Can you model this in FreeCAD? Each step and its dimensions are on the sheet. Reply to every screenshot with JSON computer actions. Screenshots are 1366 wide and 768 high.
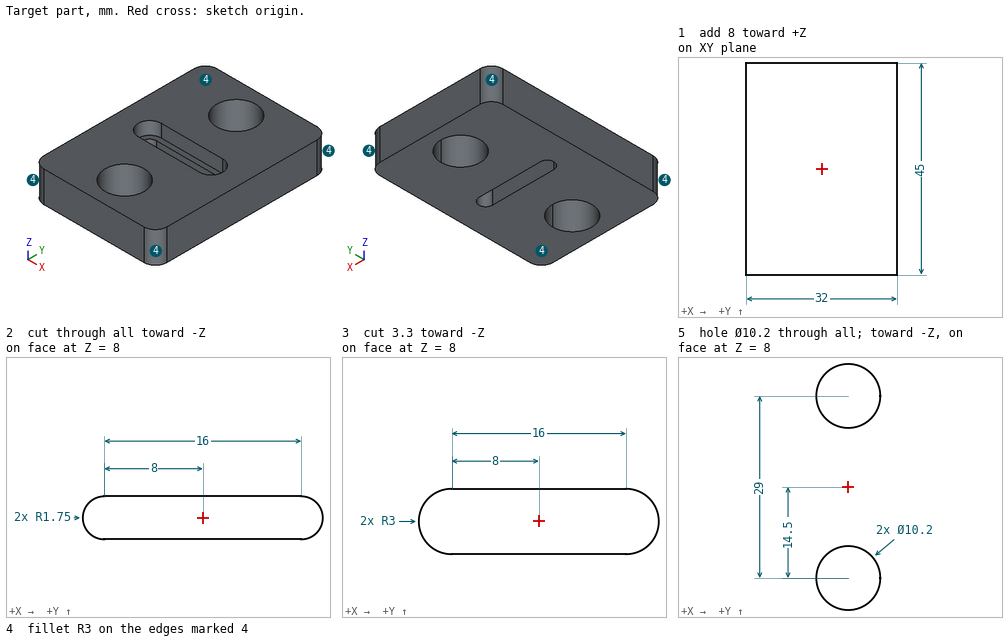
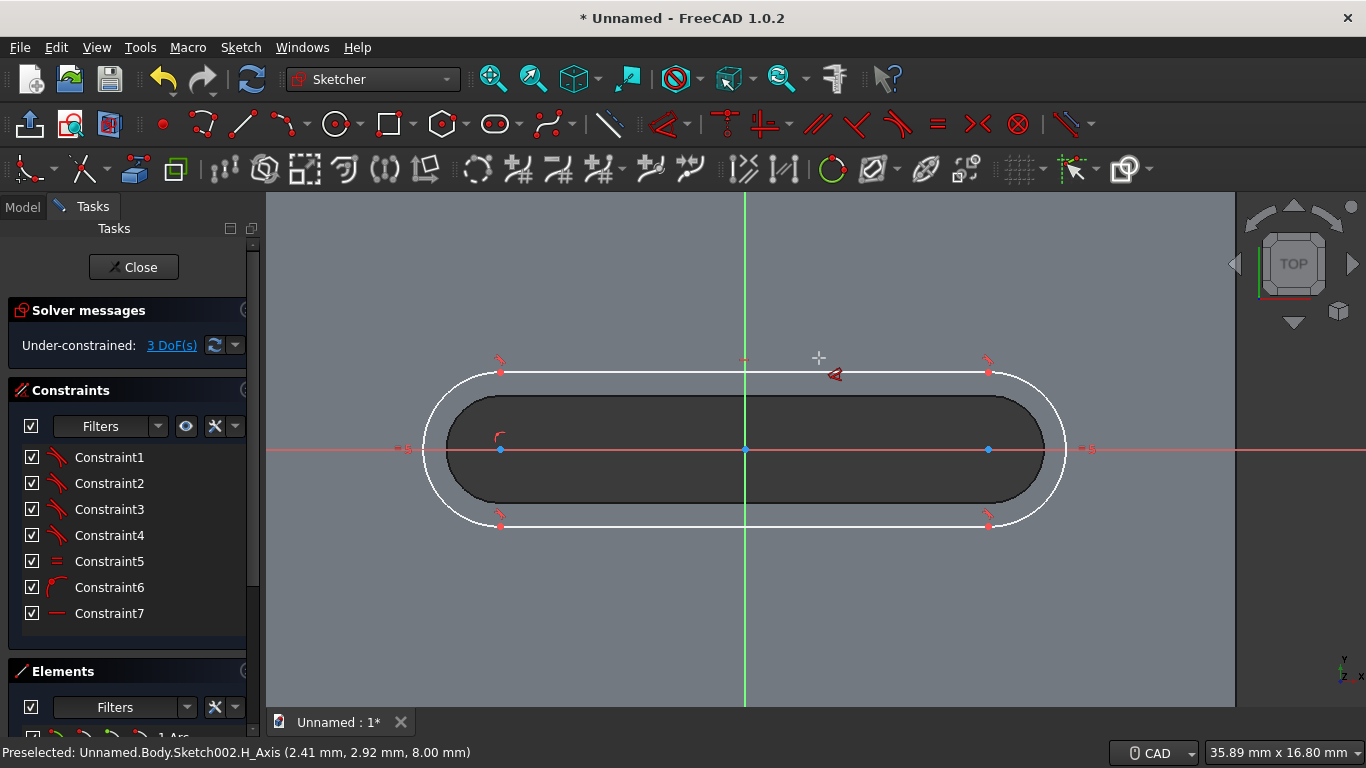
{"action": "left_click", "coordinate": [438, 404]}
{"action": "left_click", "coordinate": [412, 385]}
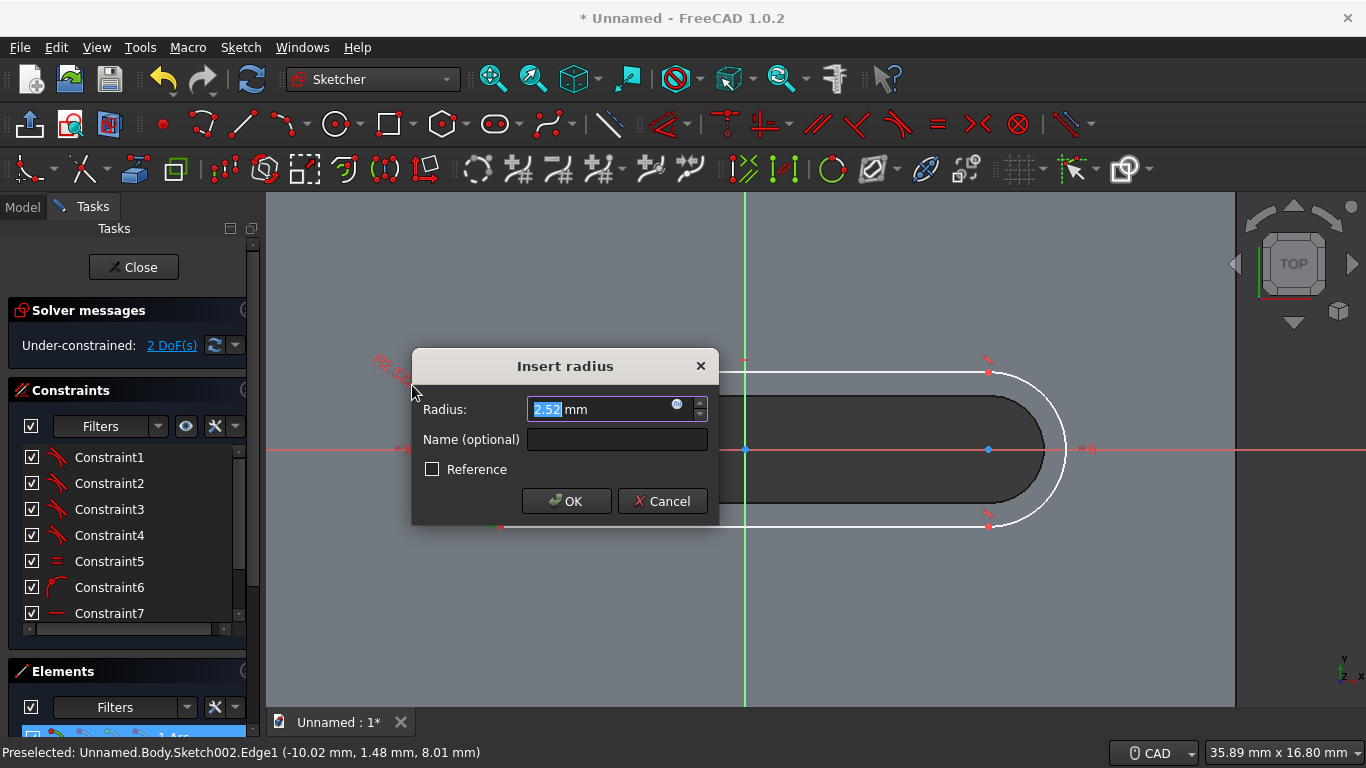
{"action": "type", "text": "3"}
{"action": "key", "text": "Return"}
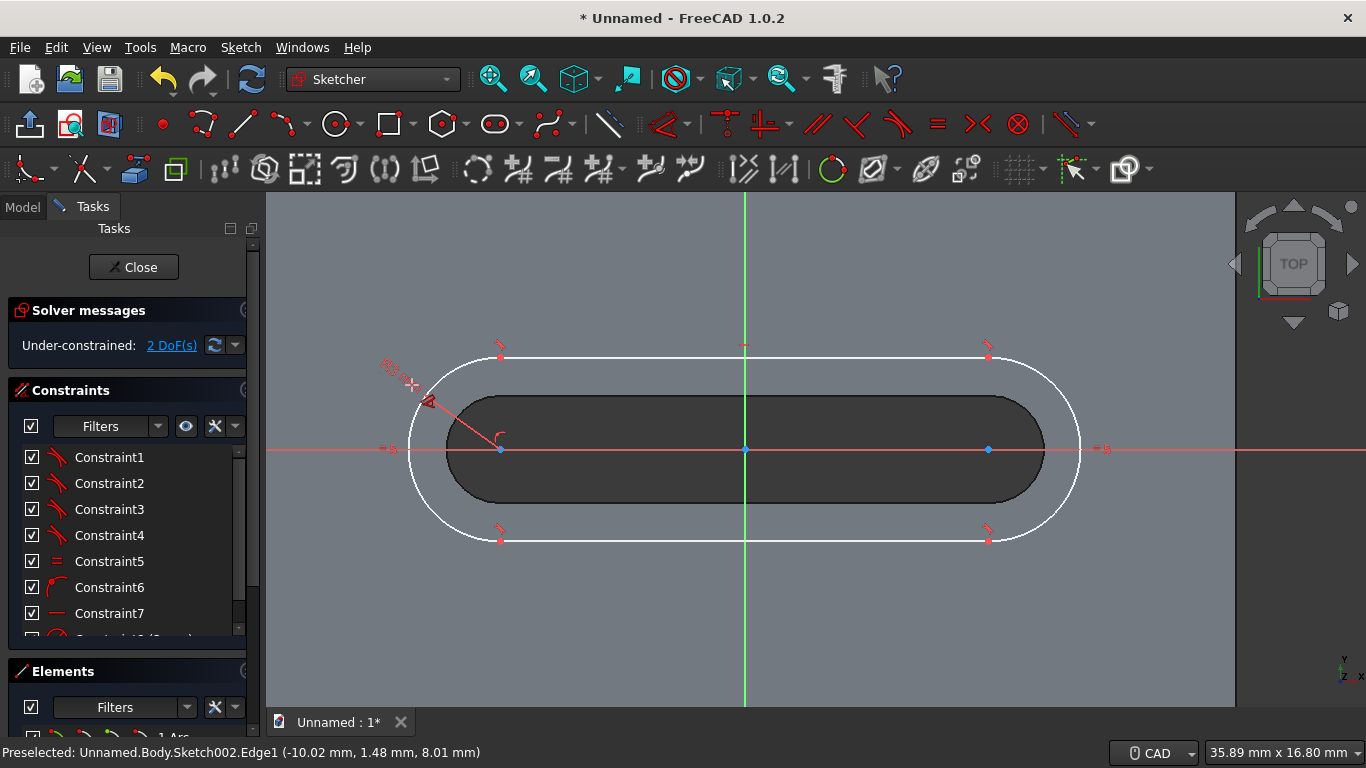
{"action": "left_click", "coordinate": [647, 358]}
{"action": "left_click", "coordinate": [632, 324]}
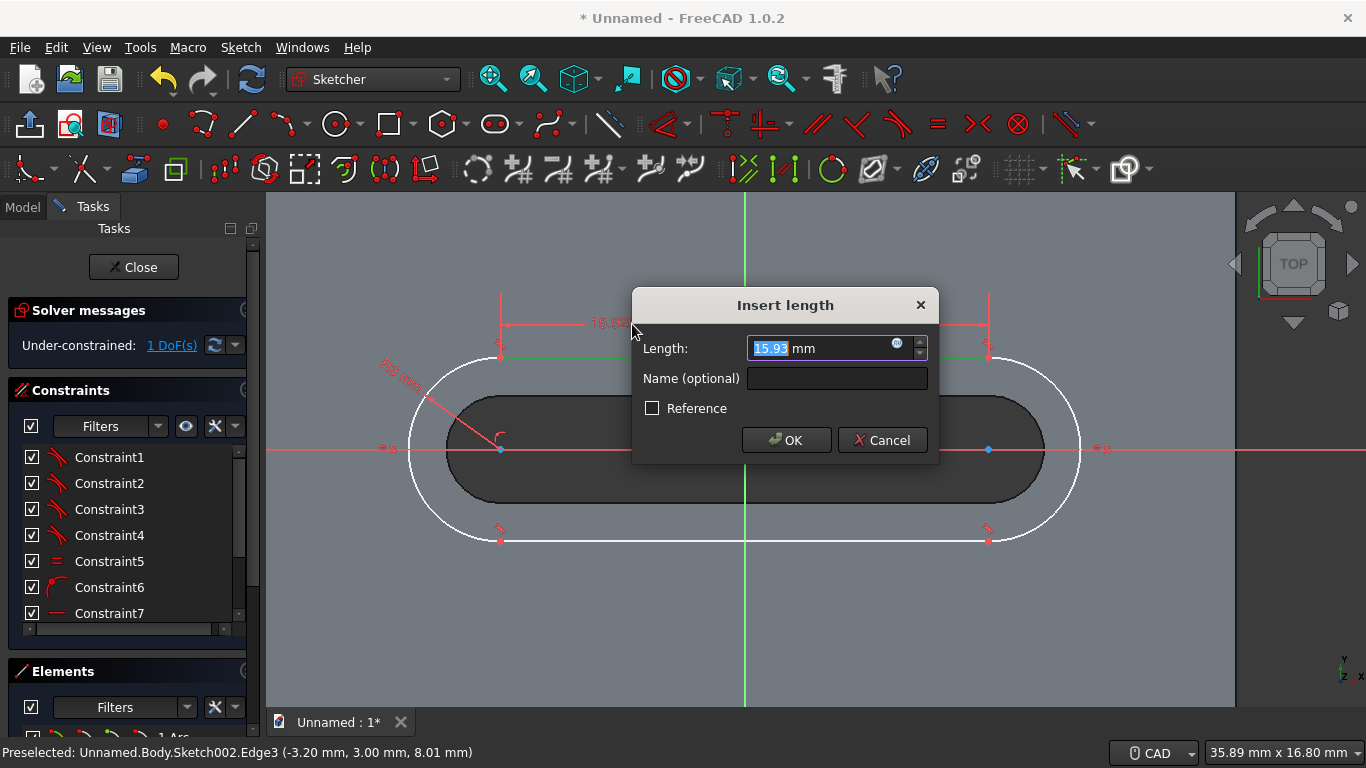
{"action": "type", "text": "16"}
{"action": "key", "text": "Return"}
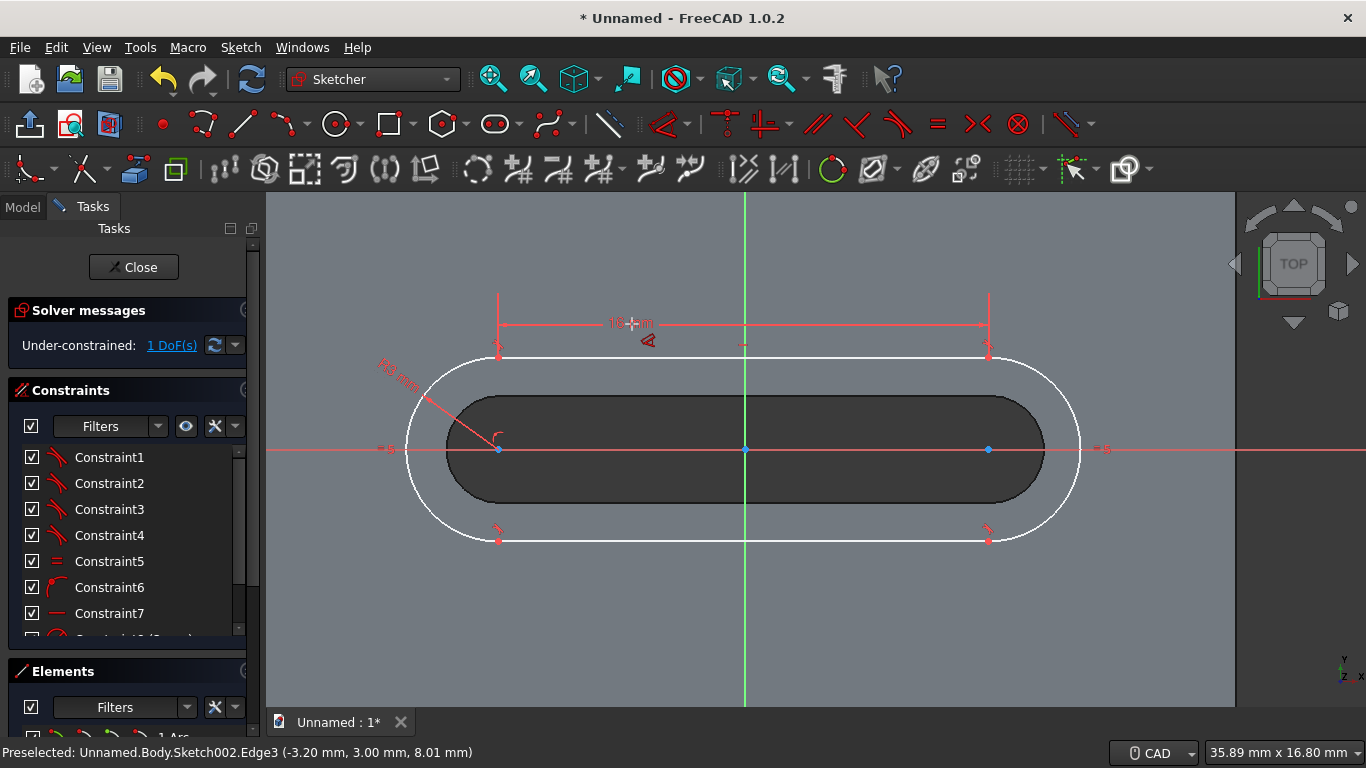
{"action": "left_click", "coordinate": [498, 358]}
{"action": "left_click", "coordinate": [535, 324]}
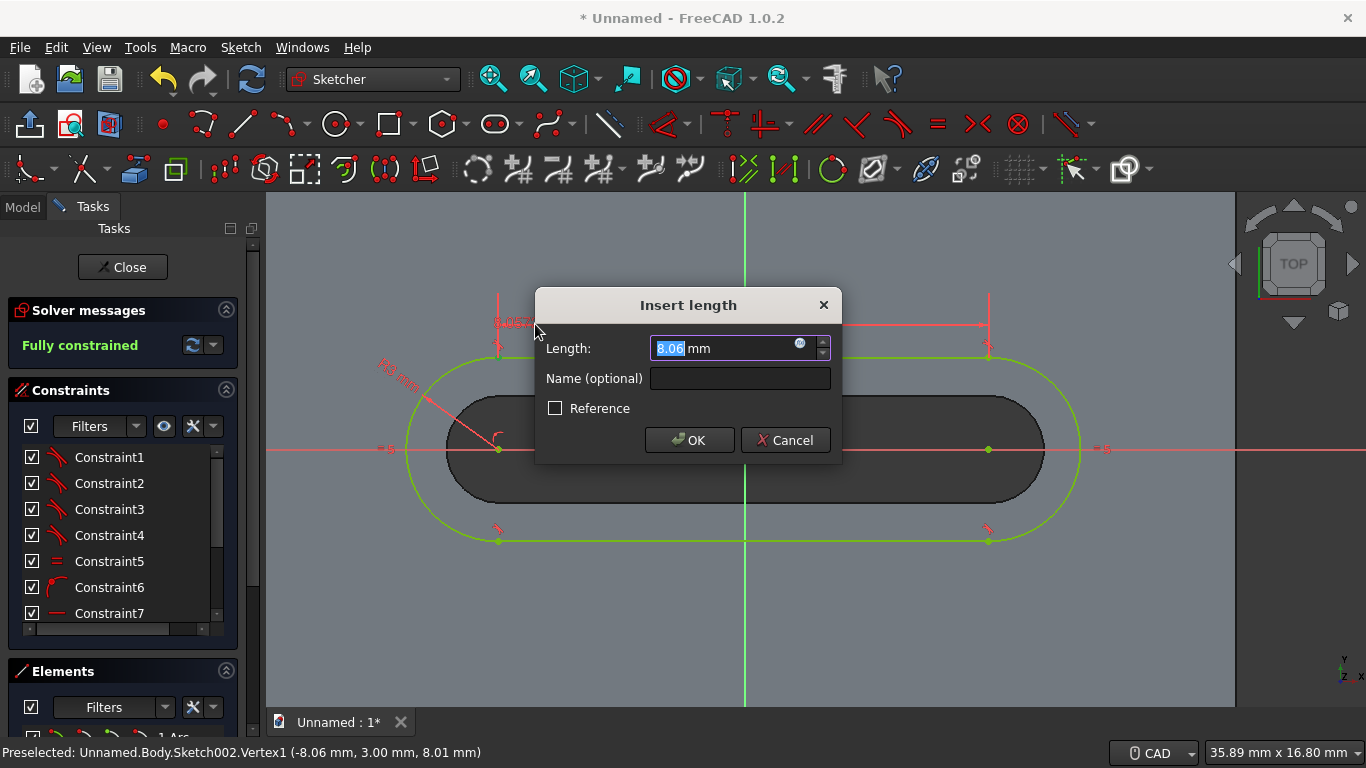
{"action": "type", "text": "8"}
{"action": "key", "text": "Return"}
{"action": "key", "text": "Escape"}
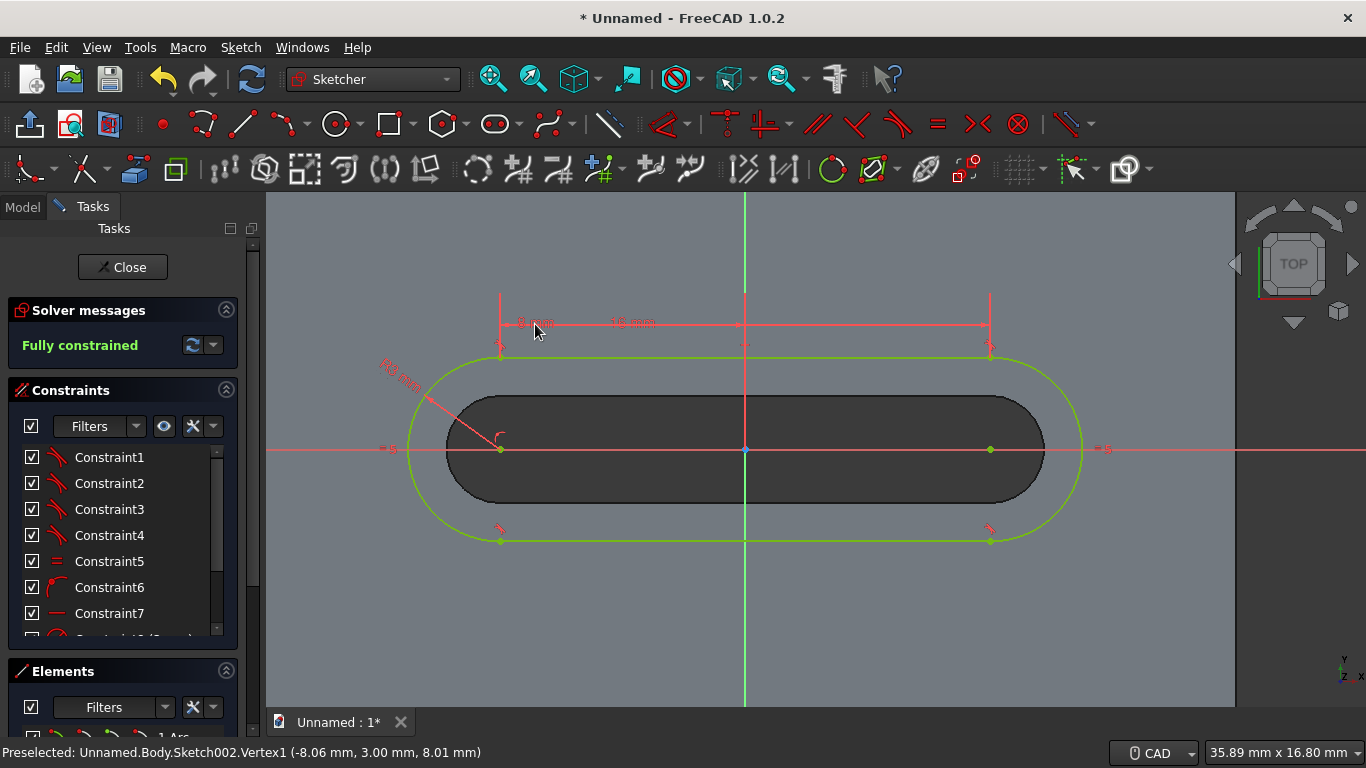
{"action": "left_click", "coordinate": [123, 267]}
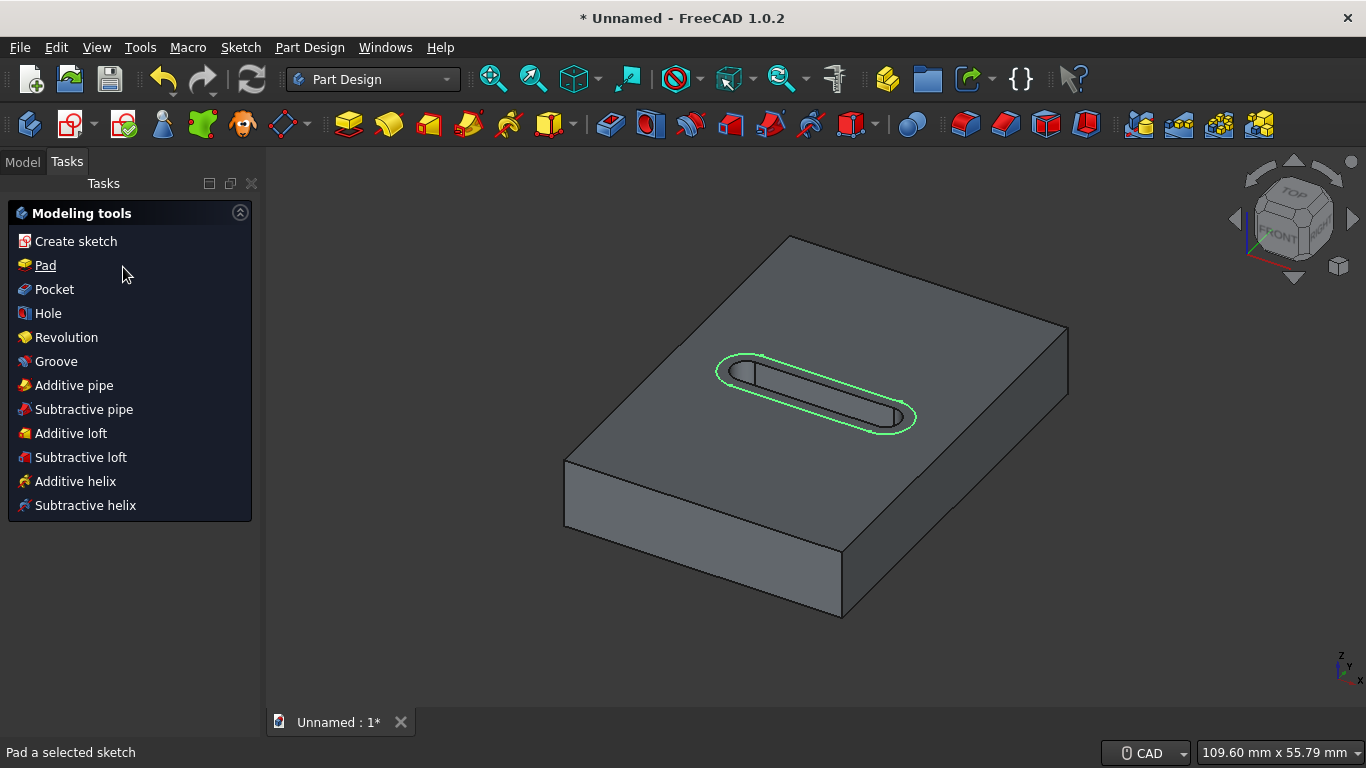
{"action": "left_click", "coordinate": [612, 124]}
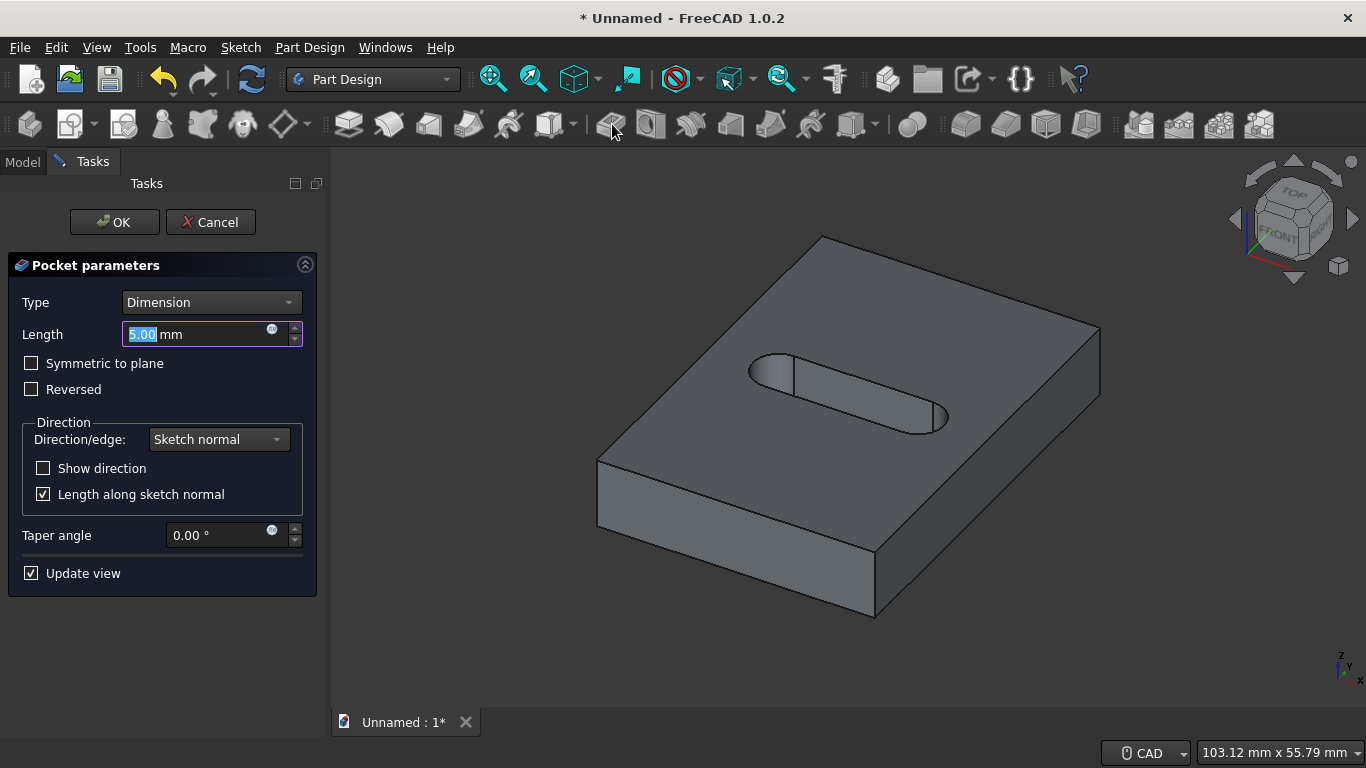
{"action": "type", "text": "3.3"}
{"action": "key", "text": "Tab"}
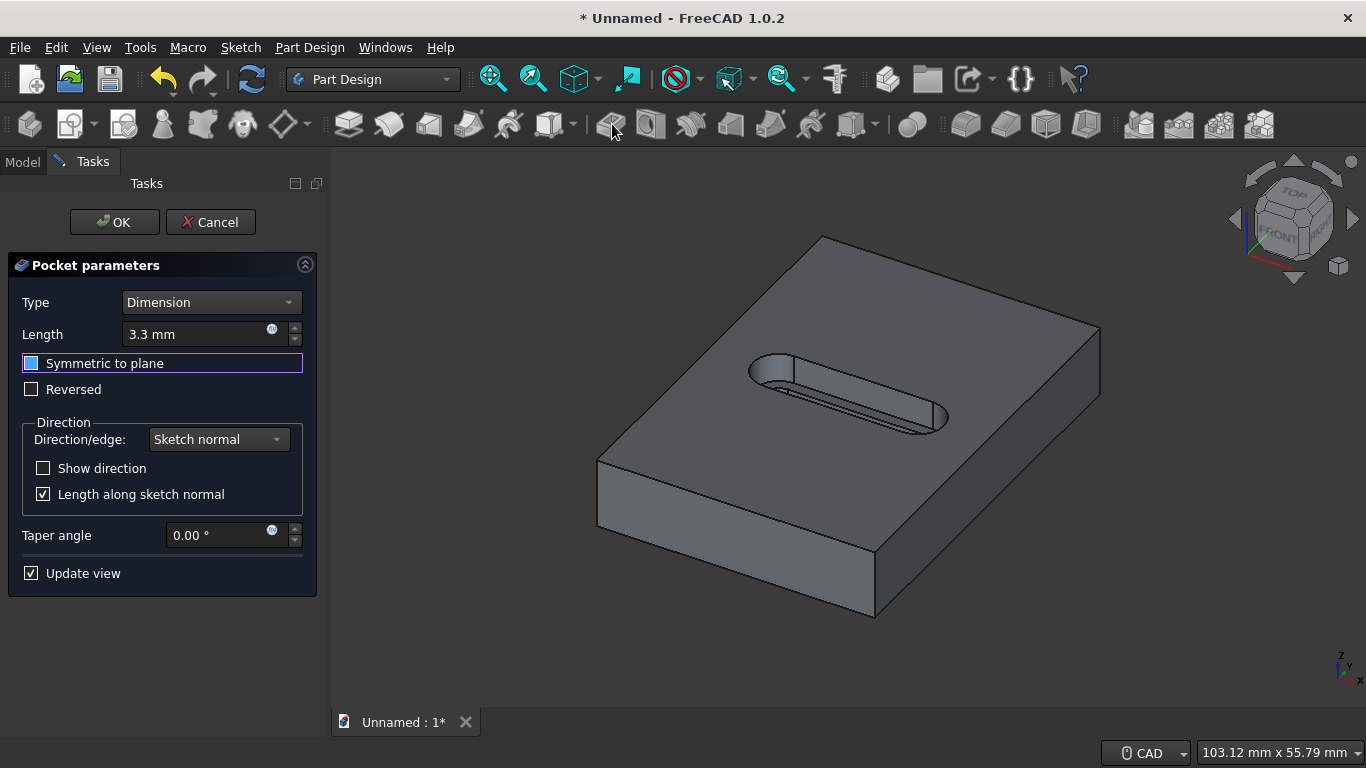
{"action": "left_click", "coordinate": [115, 222]}